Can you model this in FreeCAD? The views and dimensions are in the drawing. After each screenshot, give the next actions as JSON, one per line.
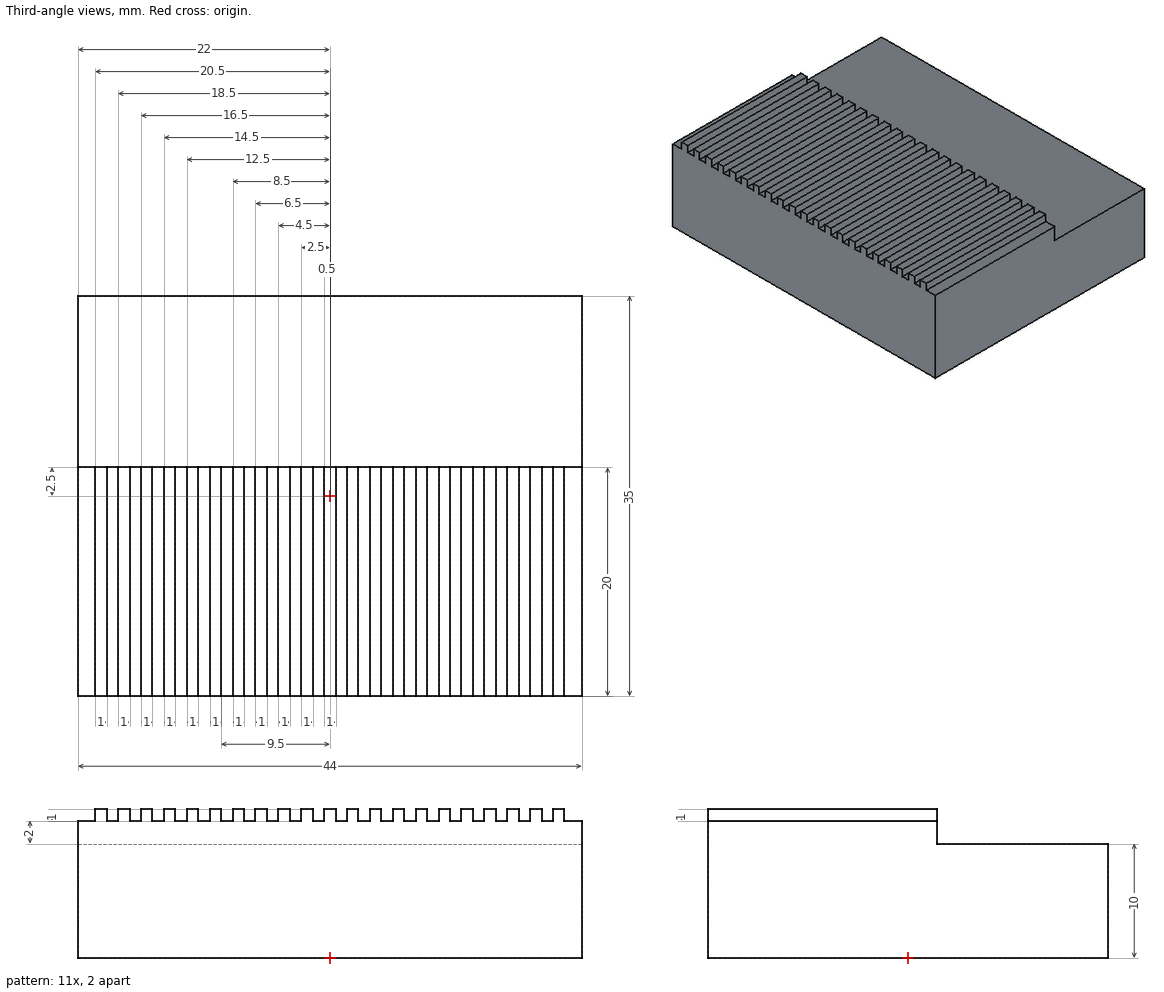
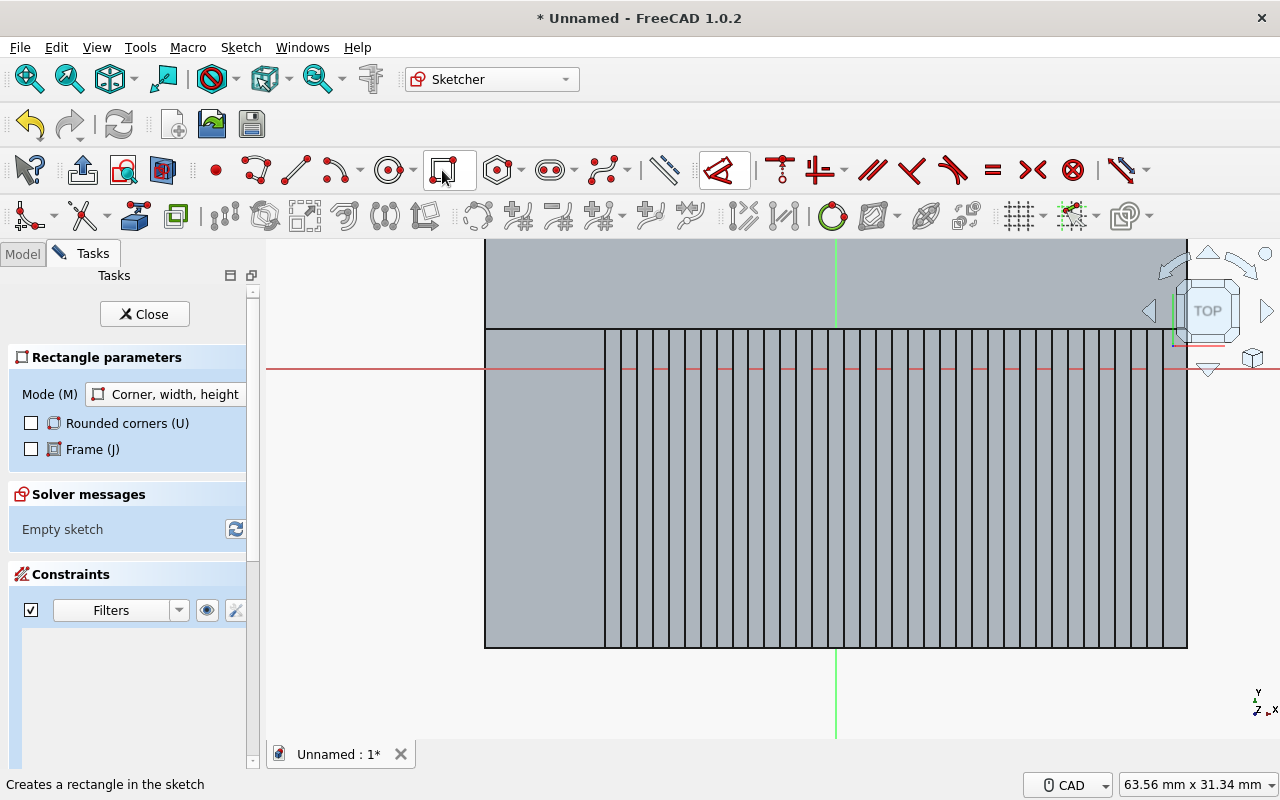
{"action": "left_click", "coordinate": [573, 329]}
{"action": "mouse_move", "coordinate": [589, 648]}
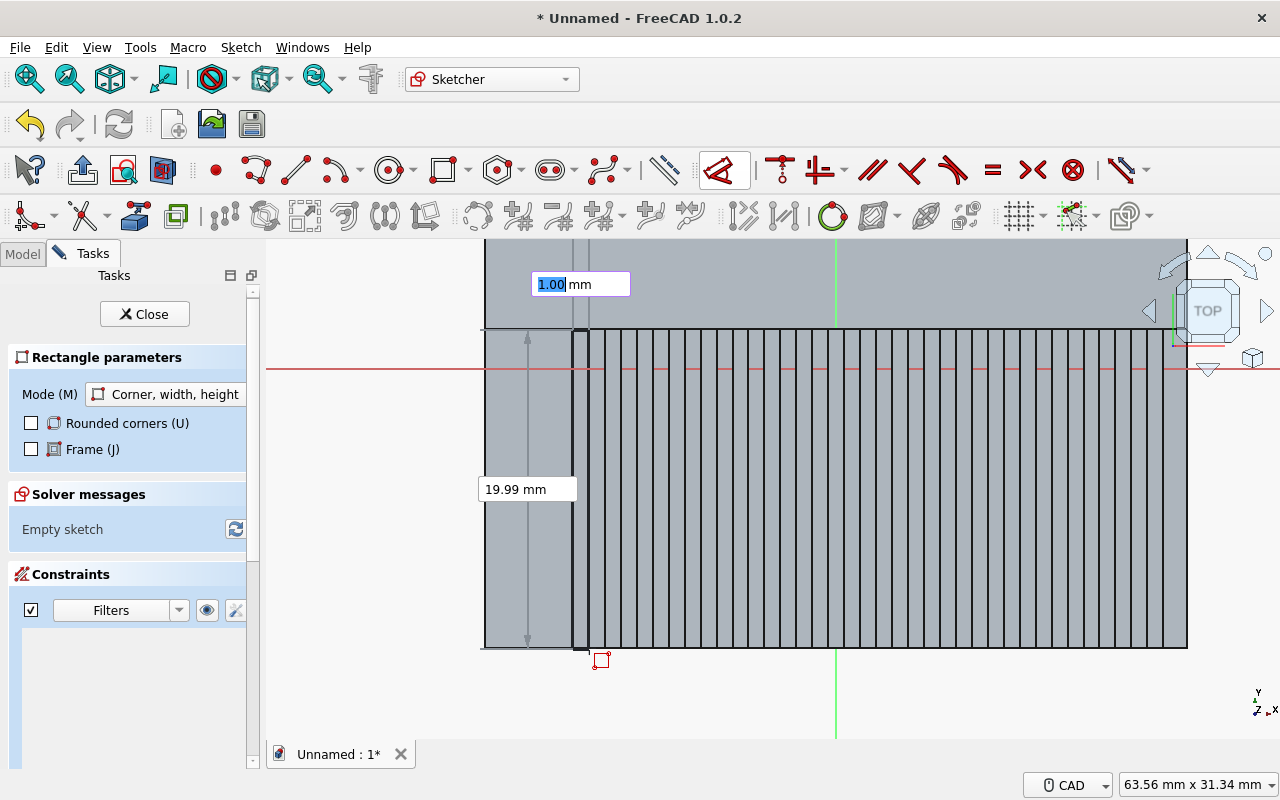
{"action": "type", "text": "1"}
{"action": "key", "text": "Tab"}
{"action": "type", "text": "20"}
{"action": "key", "text": "Return"}
{"action": "key", "text": "Escape"}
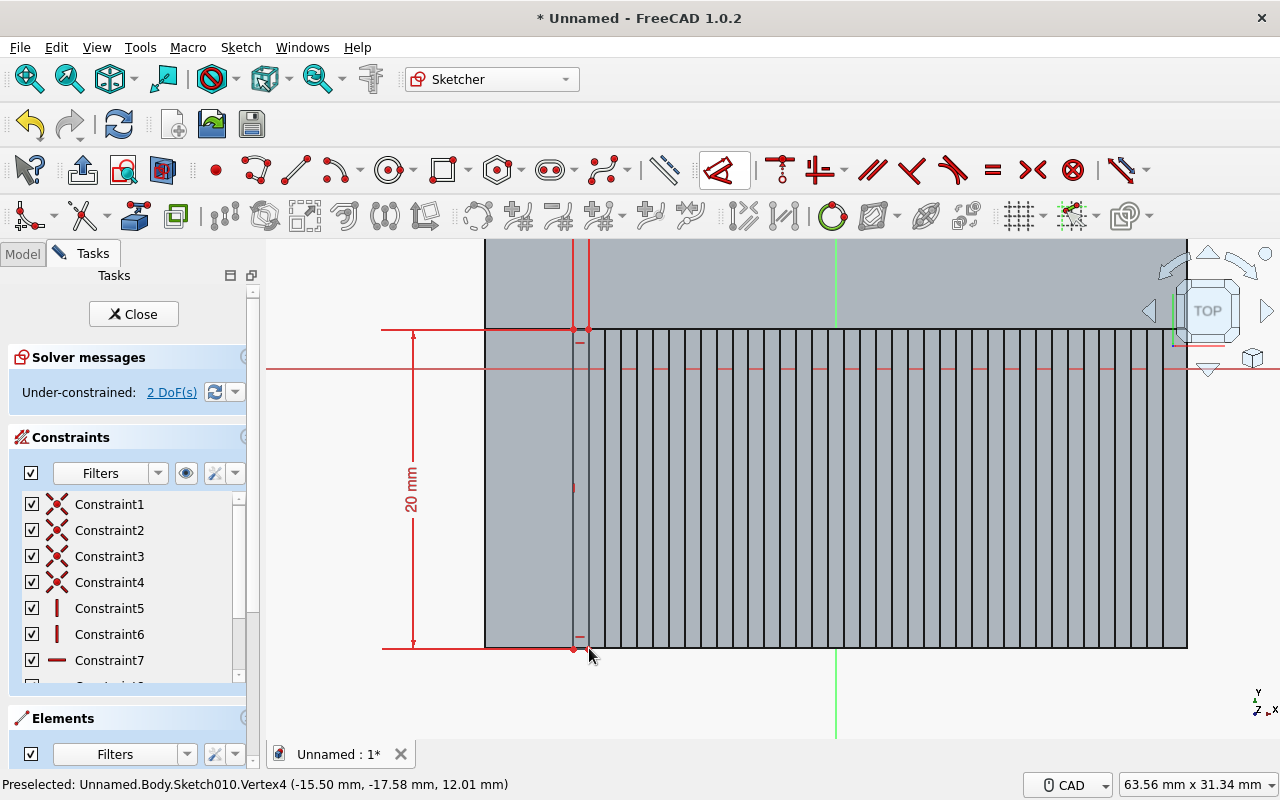
{"action": "left_click", "coordinate": [573, 330]}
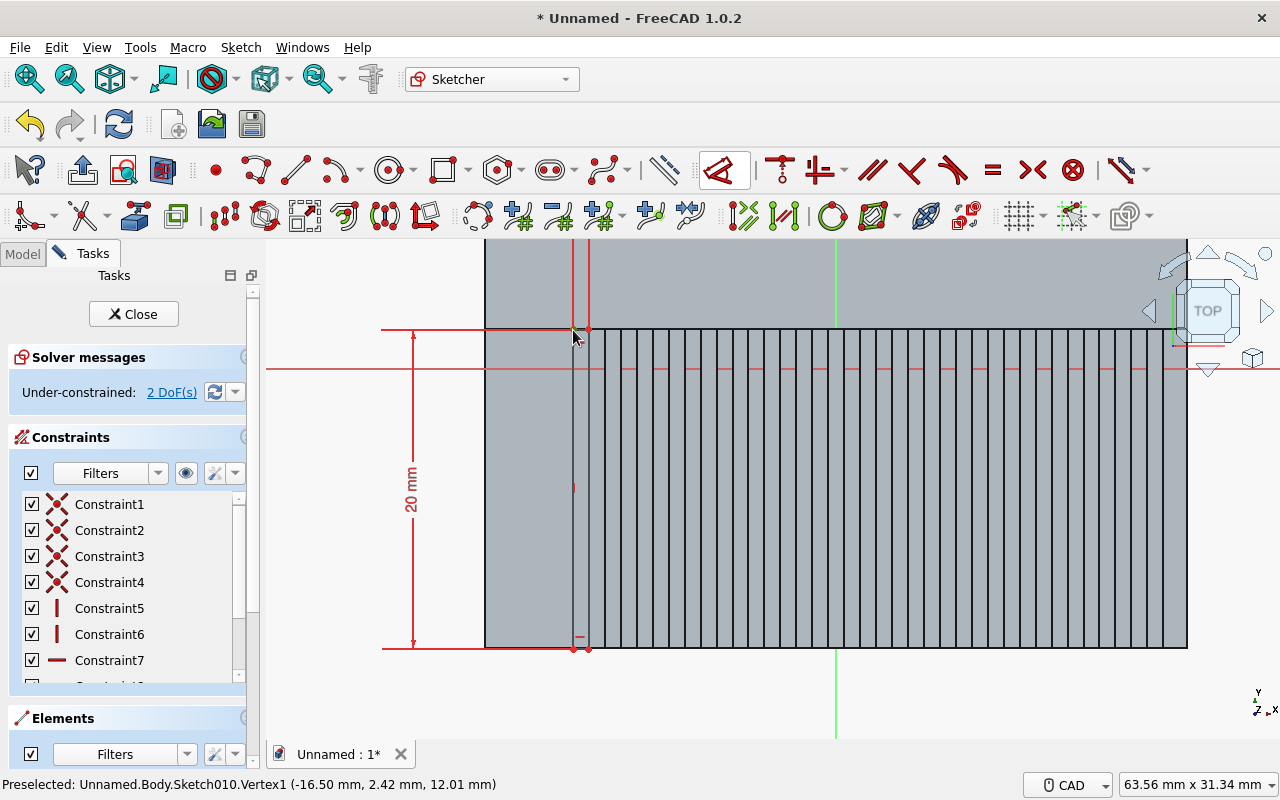
{"action": "left_click", "coordinate": [744, 170]}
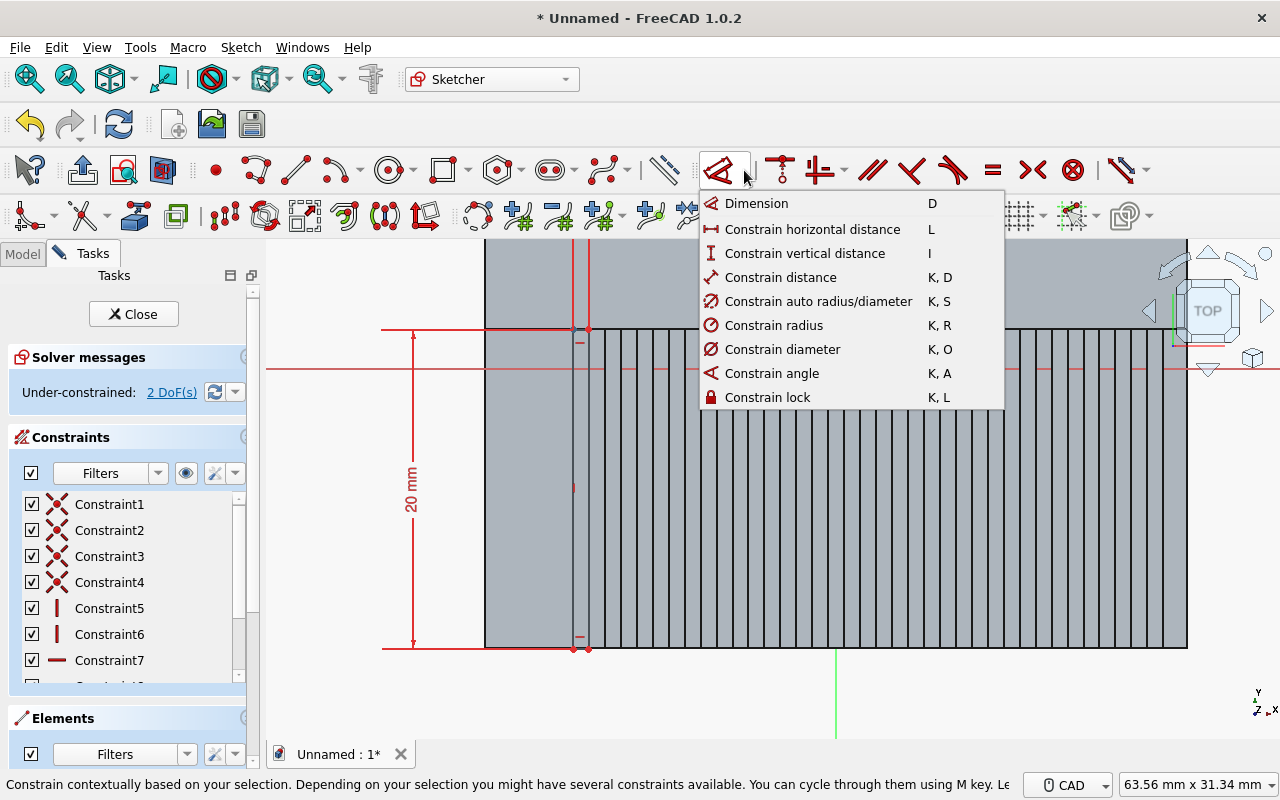
{"action": "left_click", "coordinate": [852, 253]}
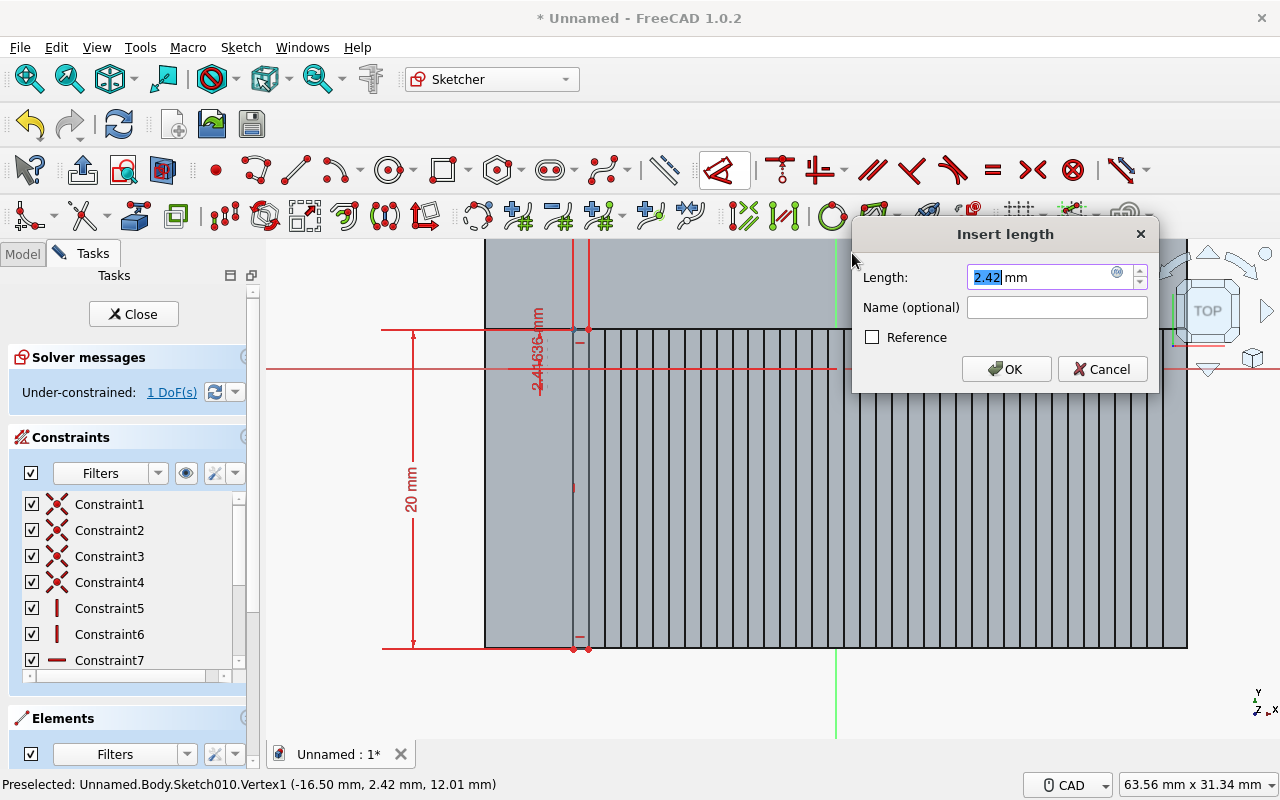
{"action": "type", "text": "2.5"}
{"action": "key", "text": "Return"}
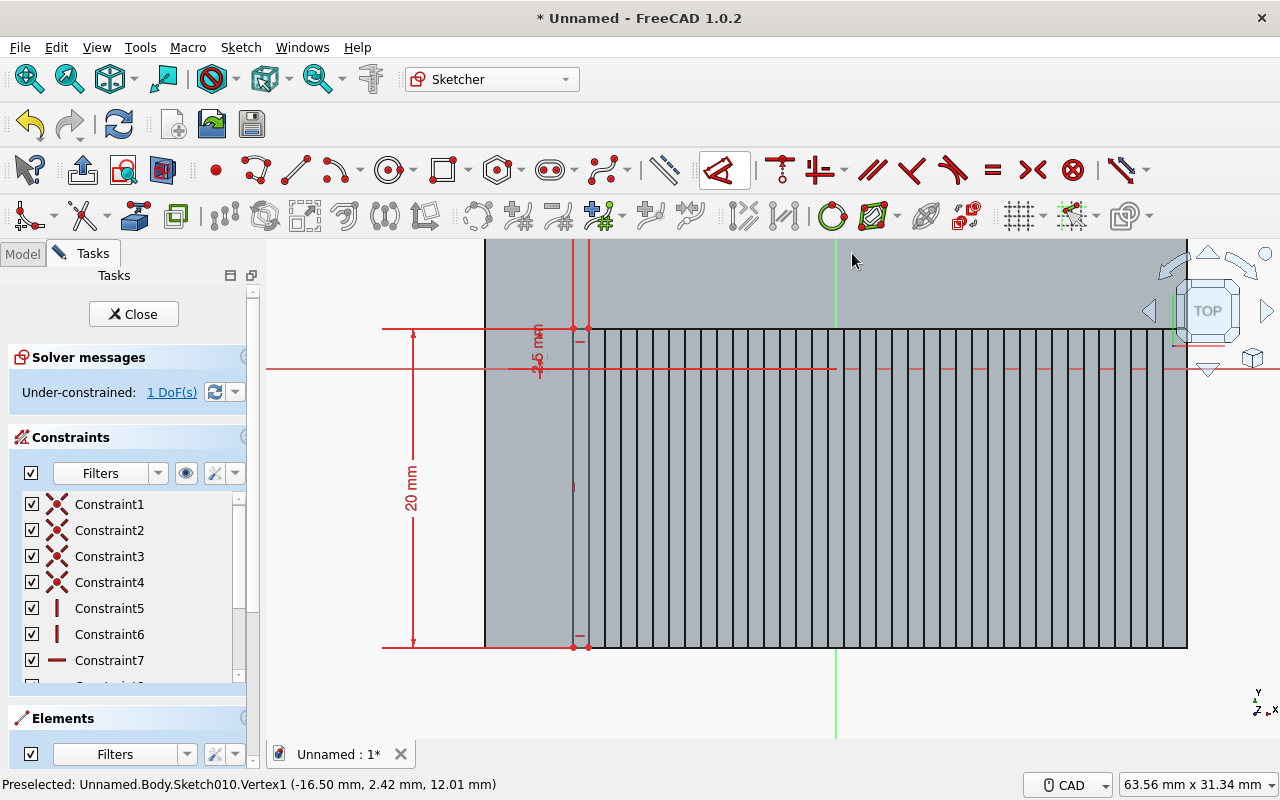
{"action": "left_click", "coordinate": [573, 329]}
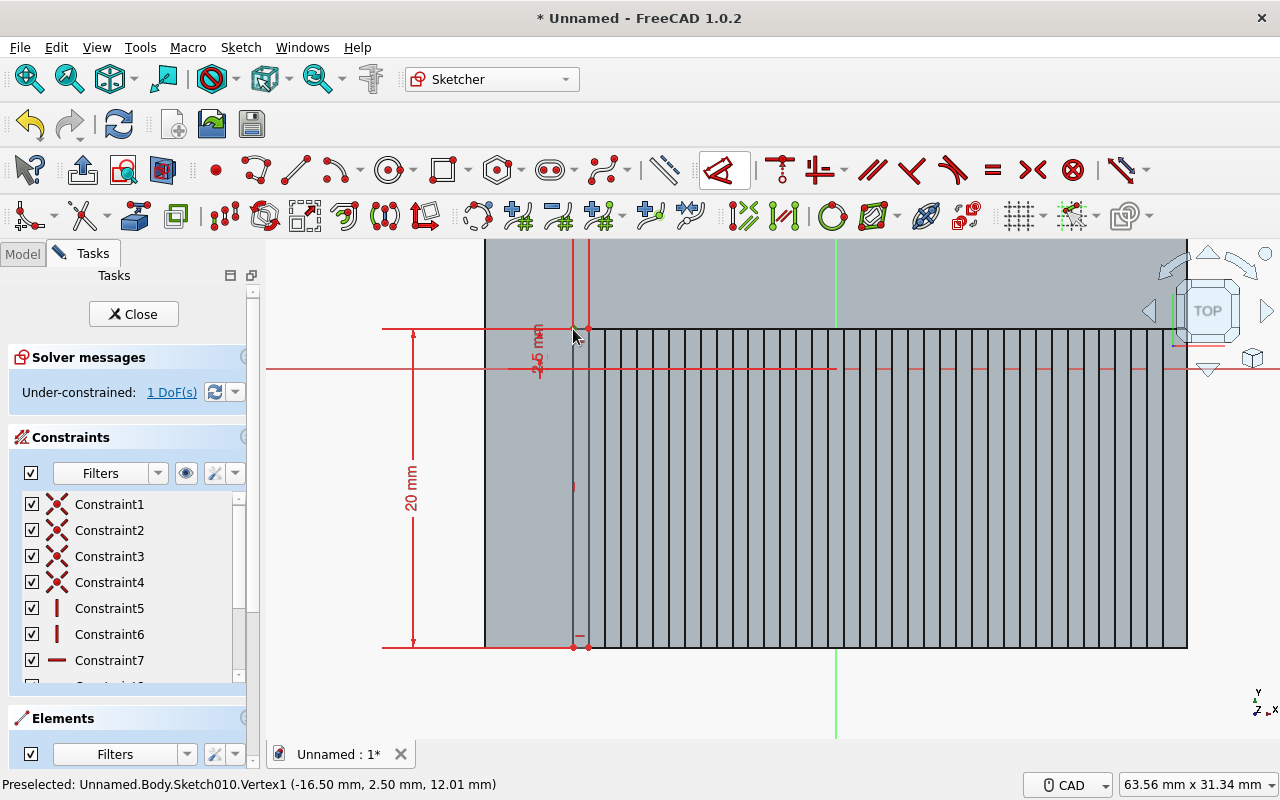
{"action": "key", "text": "l"}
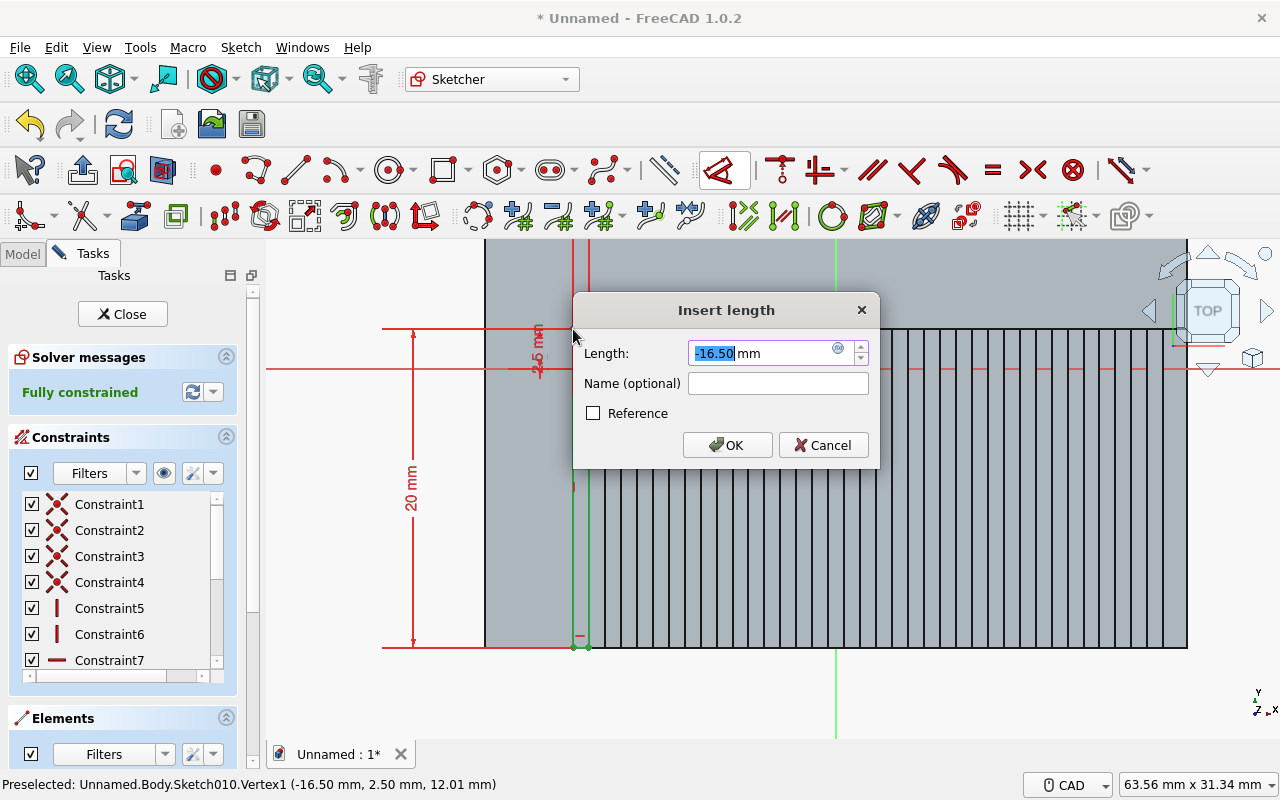
{"action": "type", "text": "-16.5"}
{"action": "key", "text": "Return"}